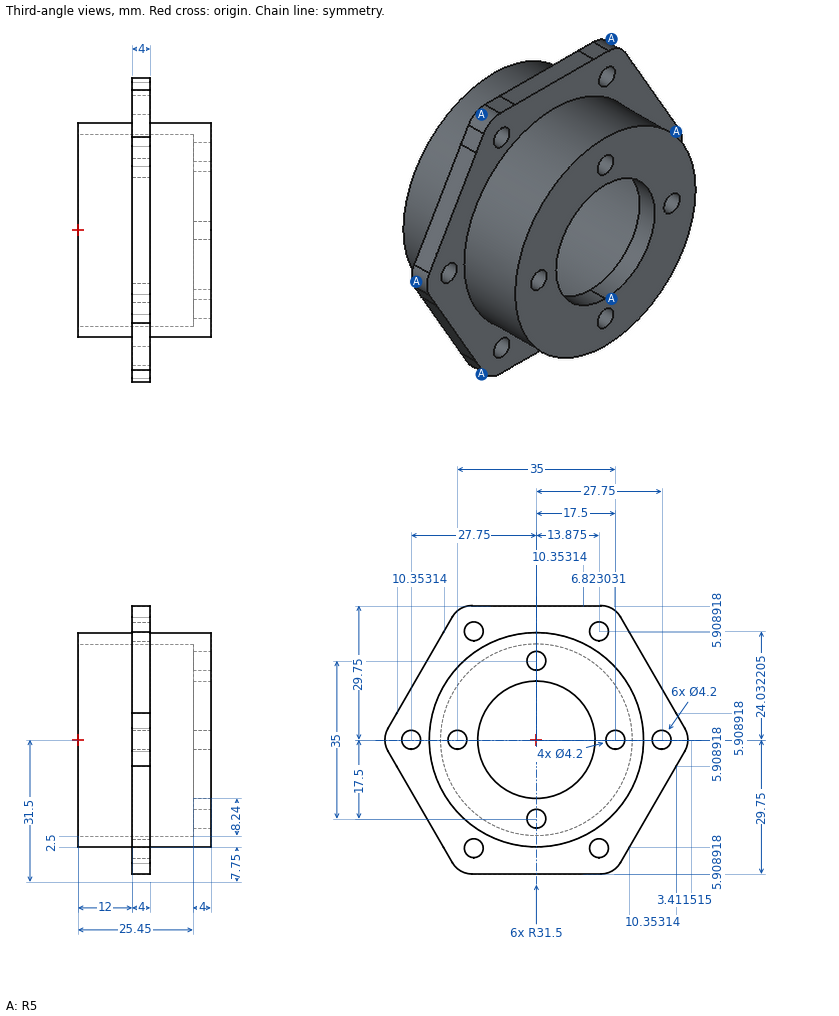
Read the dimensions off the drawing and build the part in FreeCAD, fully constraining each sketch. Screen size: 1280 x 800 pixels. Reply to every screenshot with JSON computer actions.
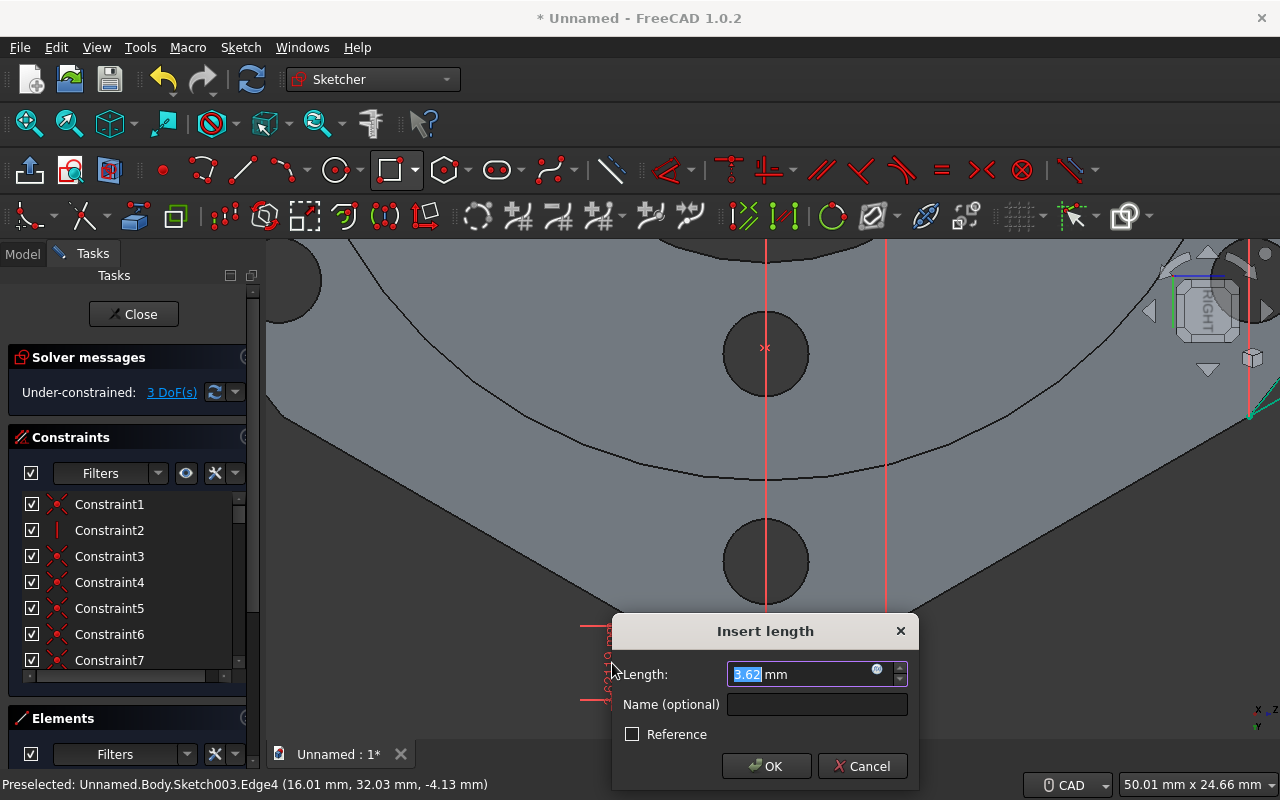
{"action": "type", "text": "3.411515"}
{"action": "key", "text": "Return"}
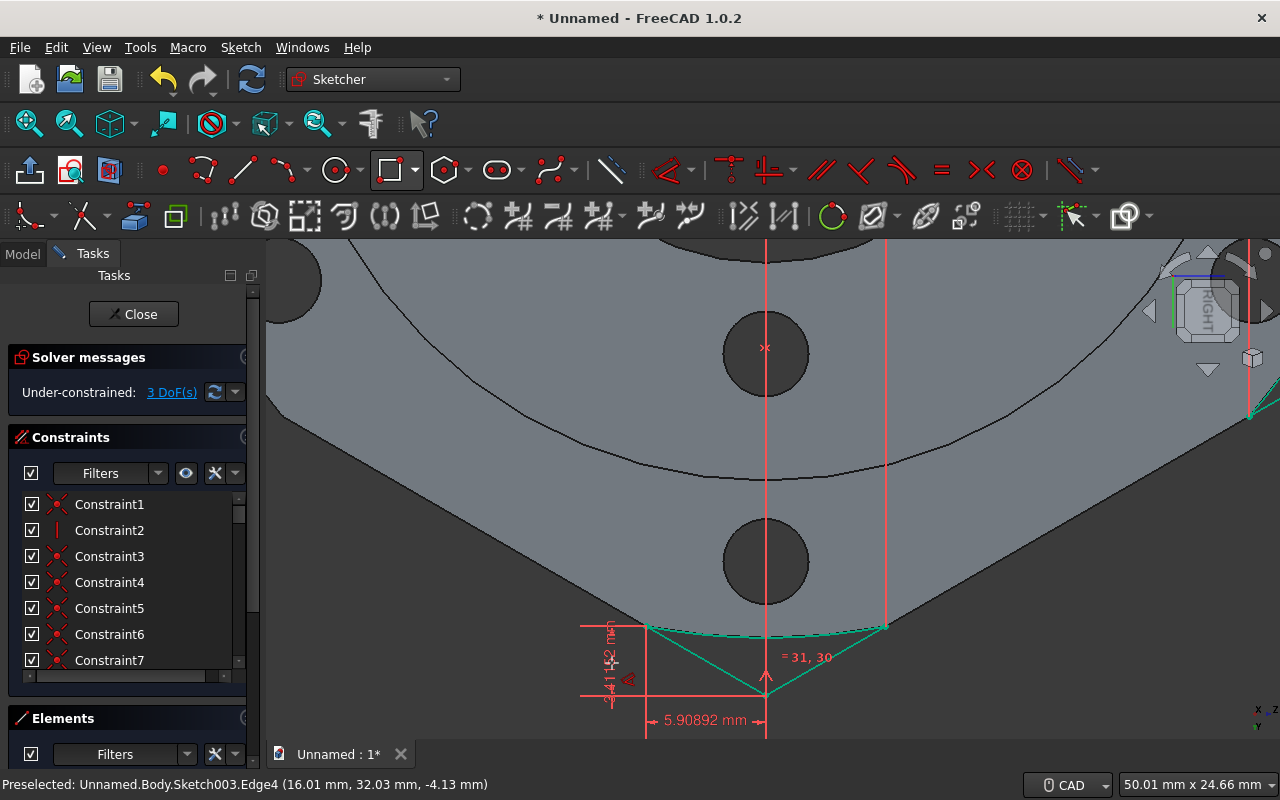
{"action": "scroll", "coordinate": [684, 649], "scroll_direction": "down", "scroll_amount": 7}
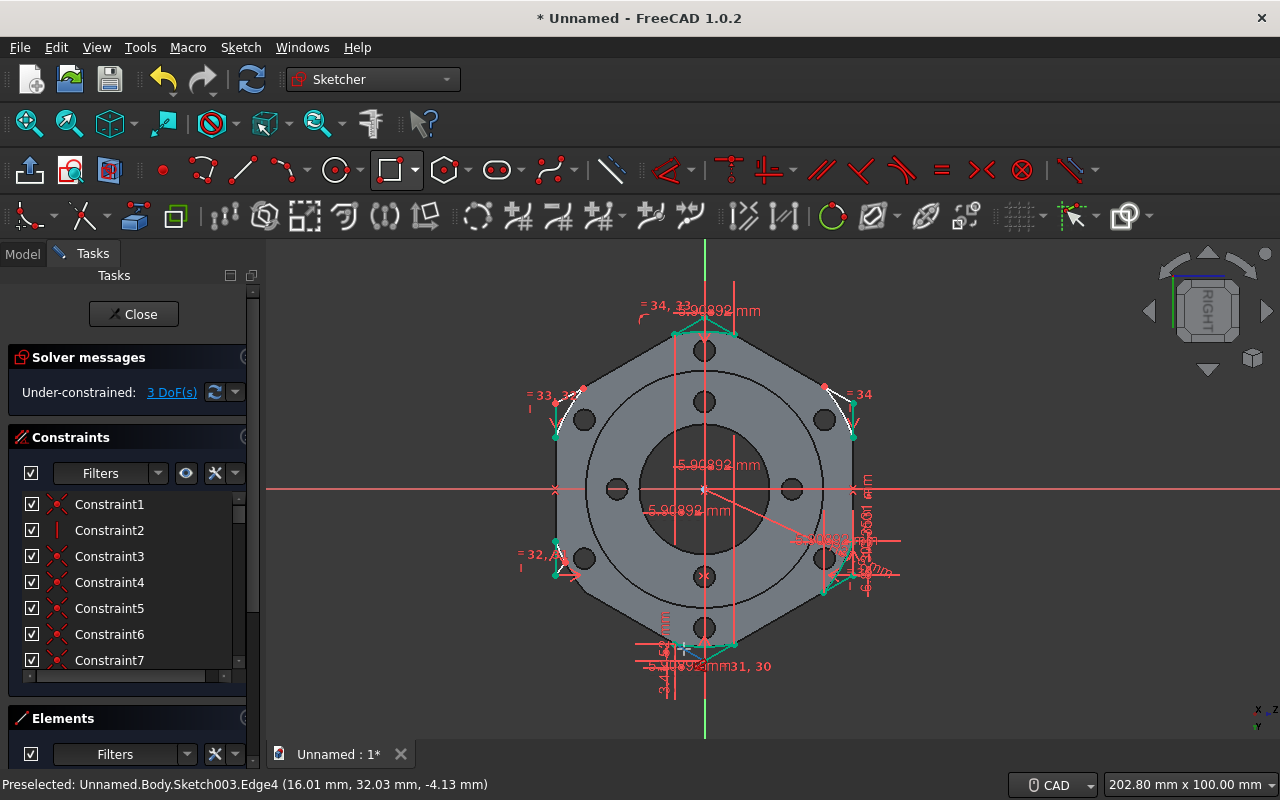
{"action": "scroll", "coordinate": [559, 571], "scroll_direction": "up", "scroll_amount": 8}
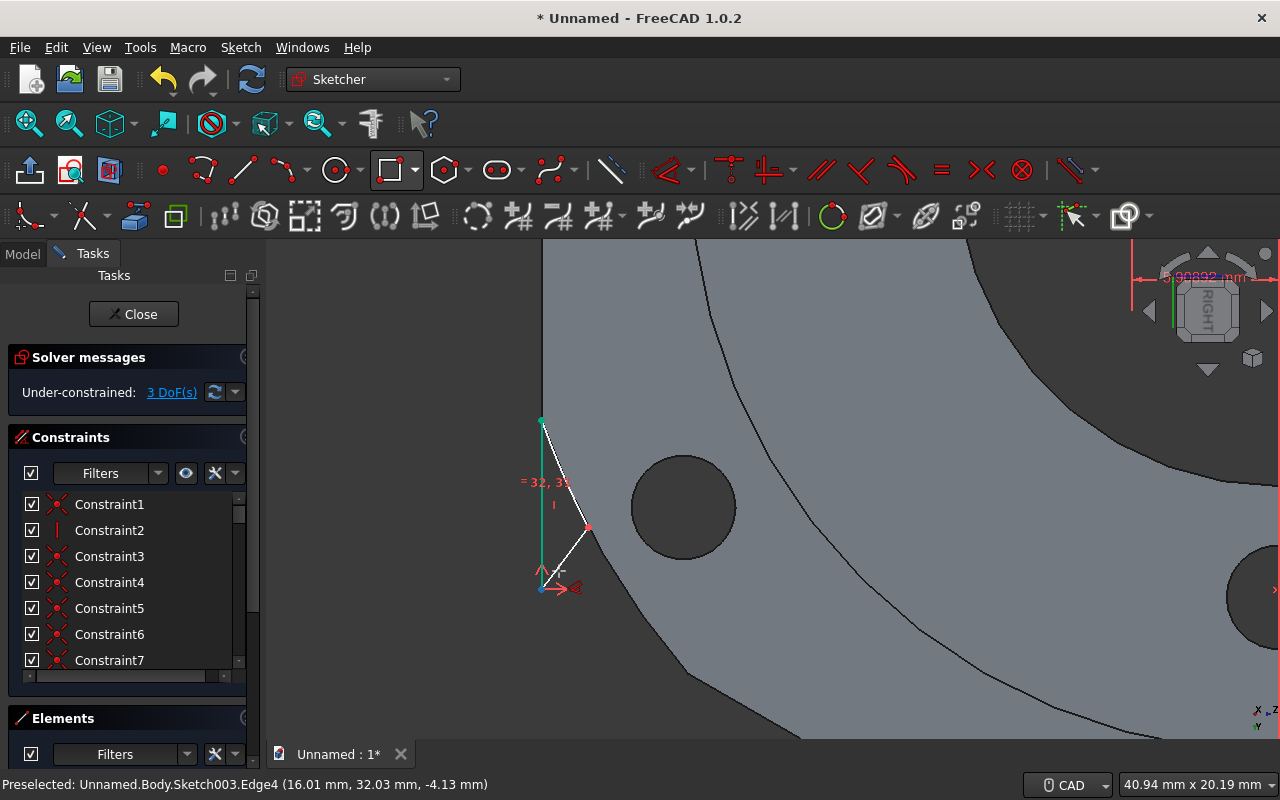
{"action": "left_click", "coordinate": [556, 571]}
{"action": "left_click", "coordinate": [565, 623]}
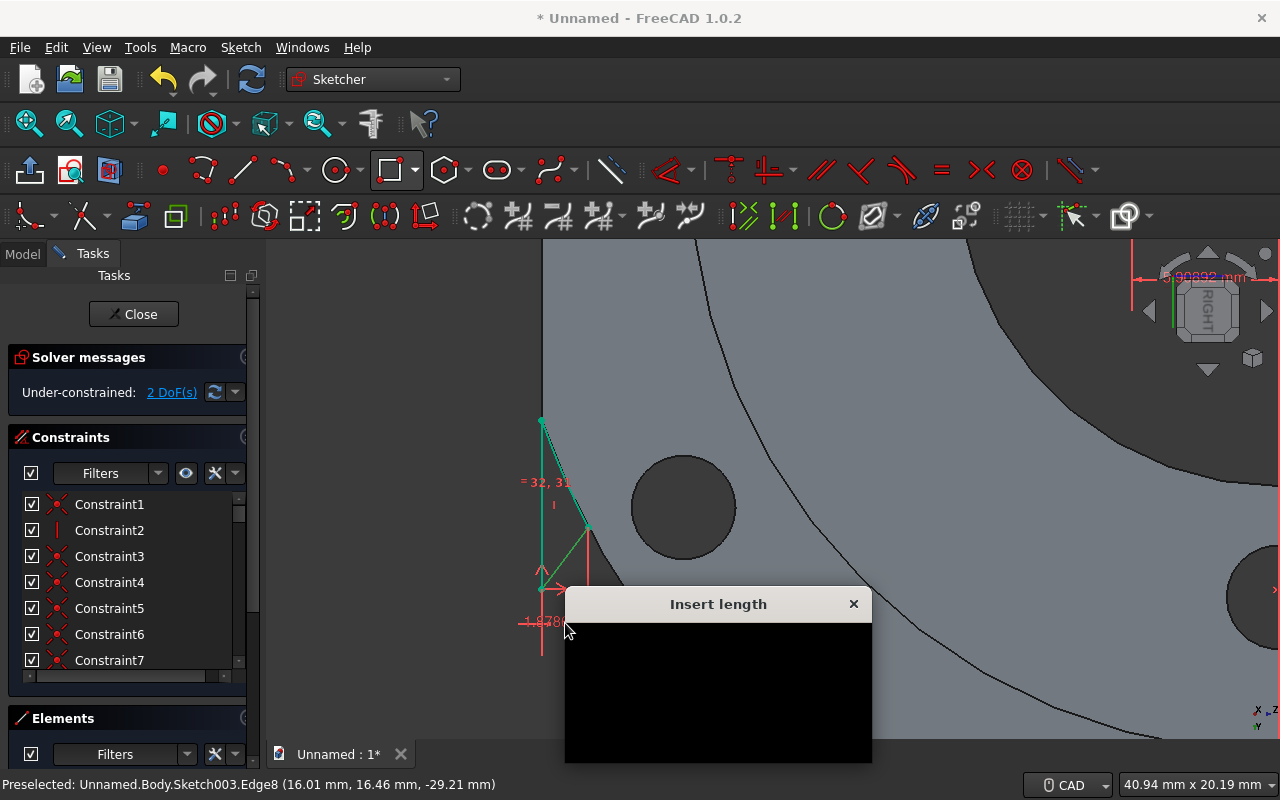
{"action": "type", "text": "5.908918"}
{"action": "key", "text": "Return"}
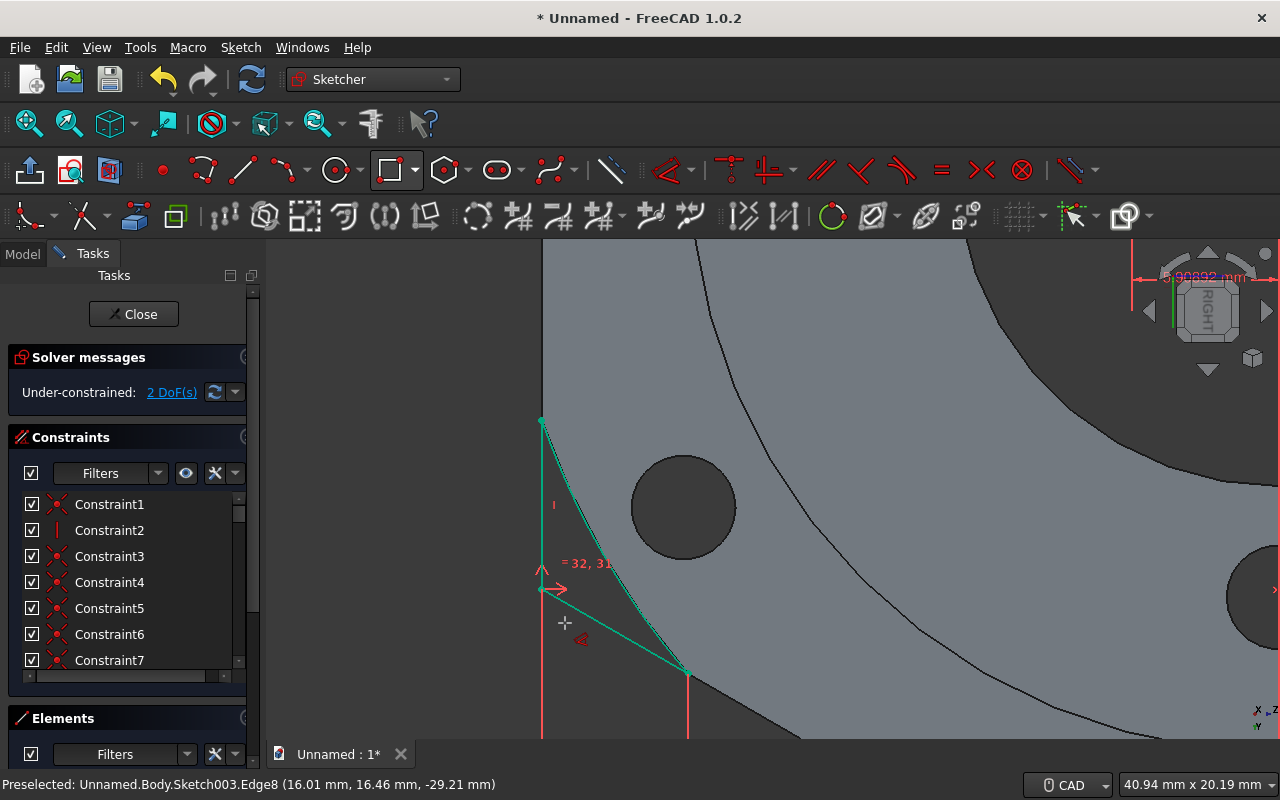
{"action": "scroll", "coordinate": [559, 571], "scroll_direction": "down", "scroll_amount": 8}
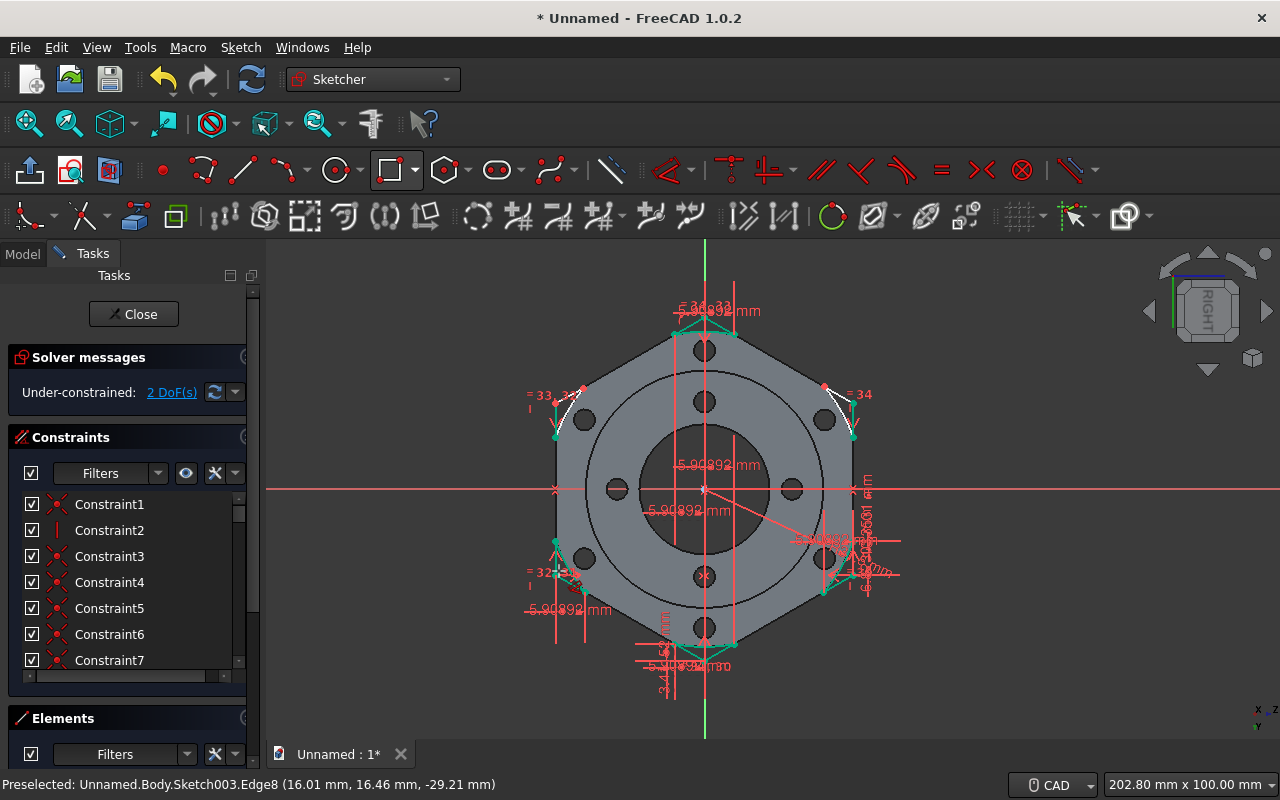
{"action": "scroll", "coordinate": [576, 393], "scroll_direction": "up", "scroll_amount": 7}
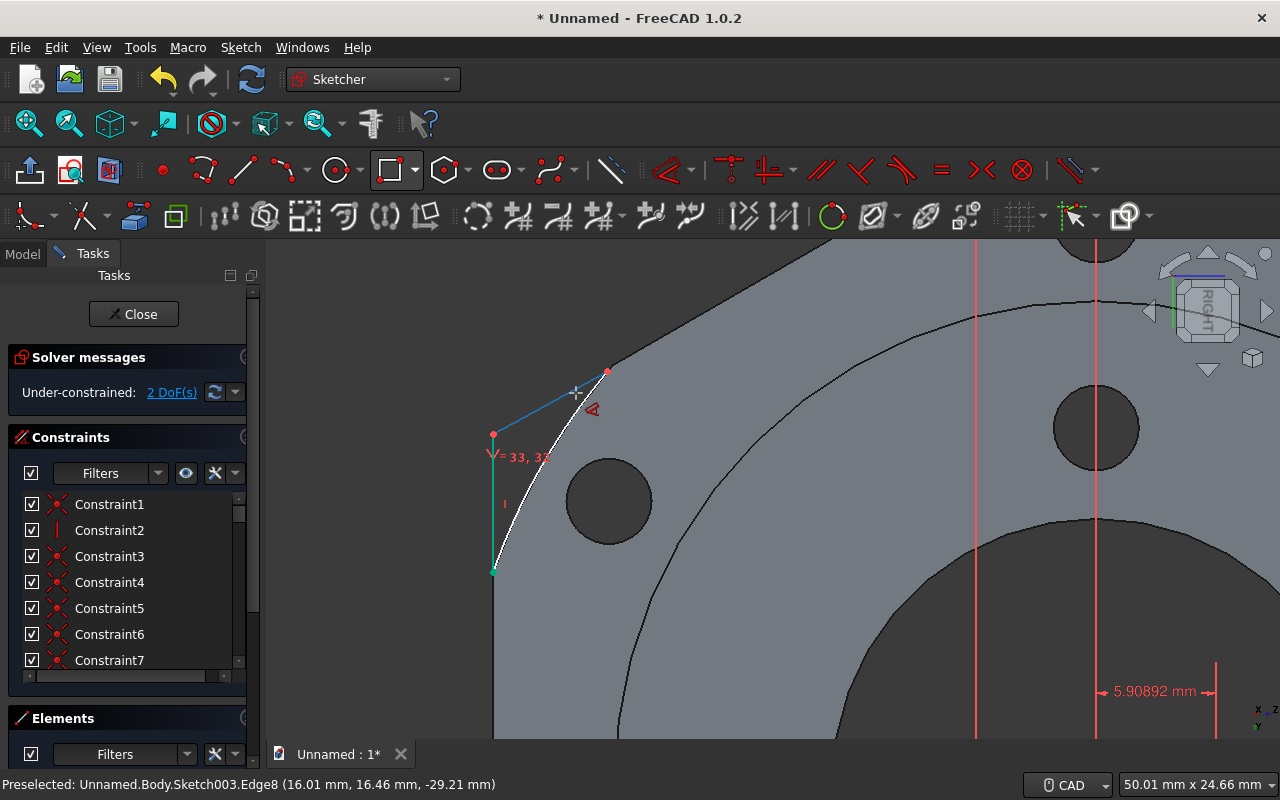
{"action": "left_click", "coordinate": [573, 391]}
{"action": "left_click", "coordinate": [550, 338]}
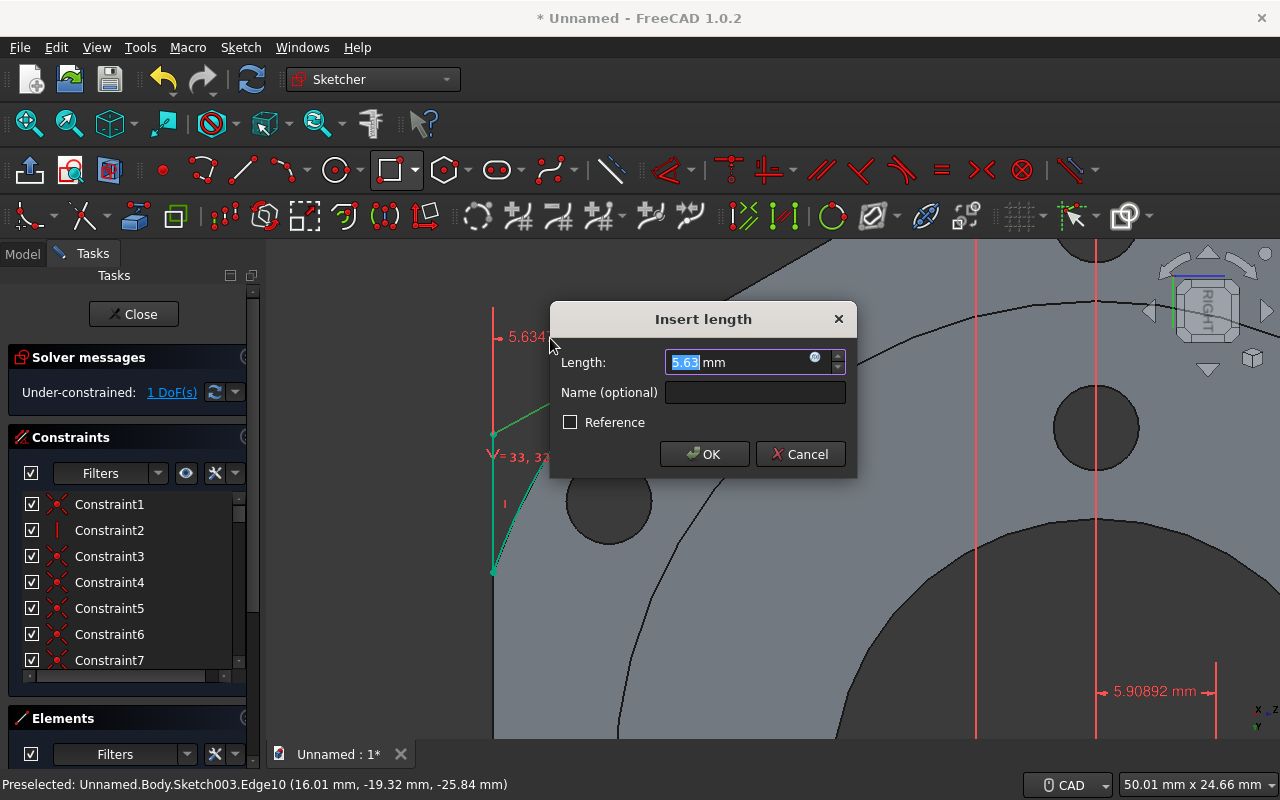
{"action": "type", "text": "5.908918"}
{"action": "key", "text": "Return"}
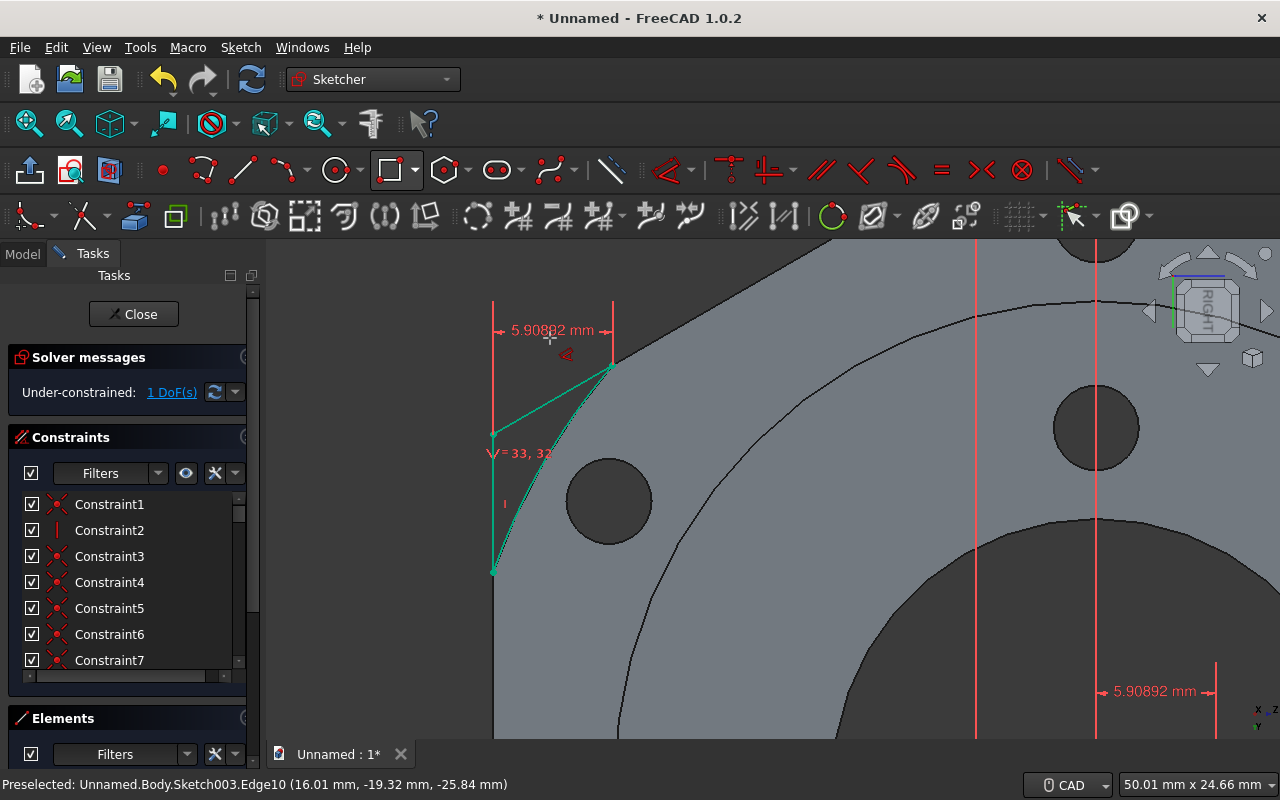
{"action": "scroll", "coordinate": [576, 393], "scroll_direction": "down", "scroll_amount": 7}